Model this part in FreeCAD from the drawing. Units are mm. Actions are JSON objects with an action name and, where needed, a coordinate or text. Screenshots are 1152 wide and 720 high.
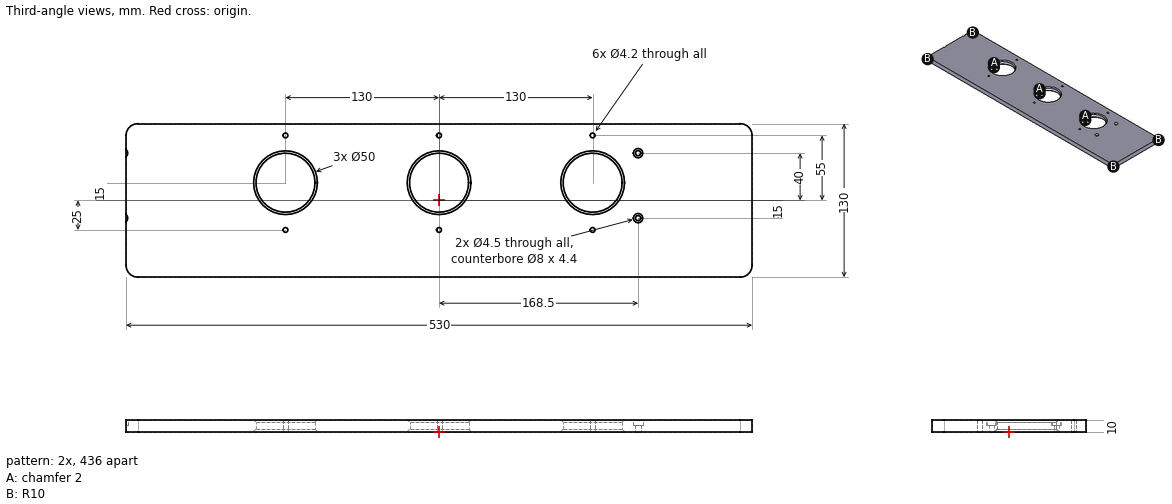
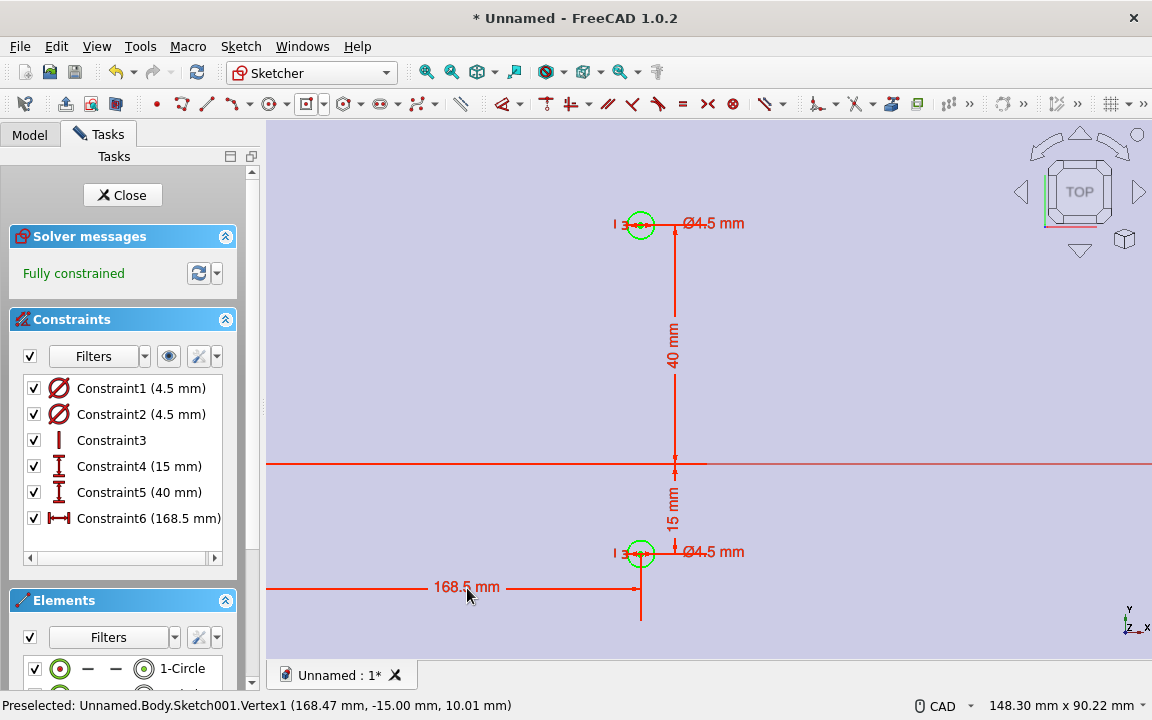
{"action": "left_click", "coordinate": [123, 195]}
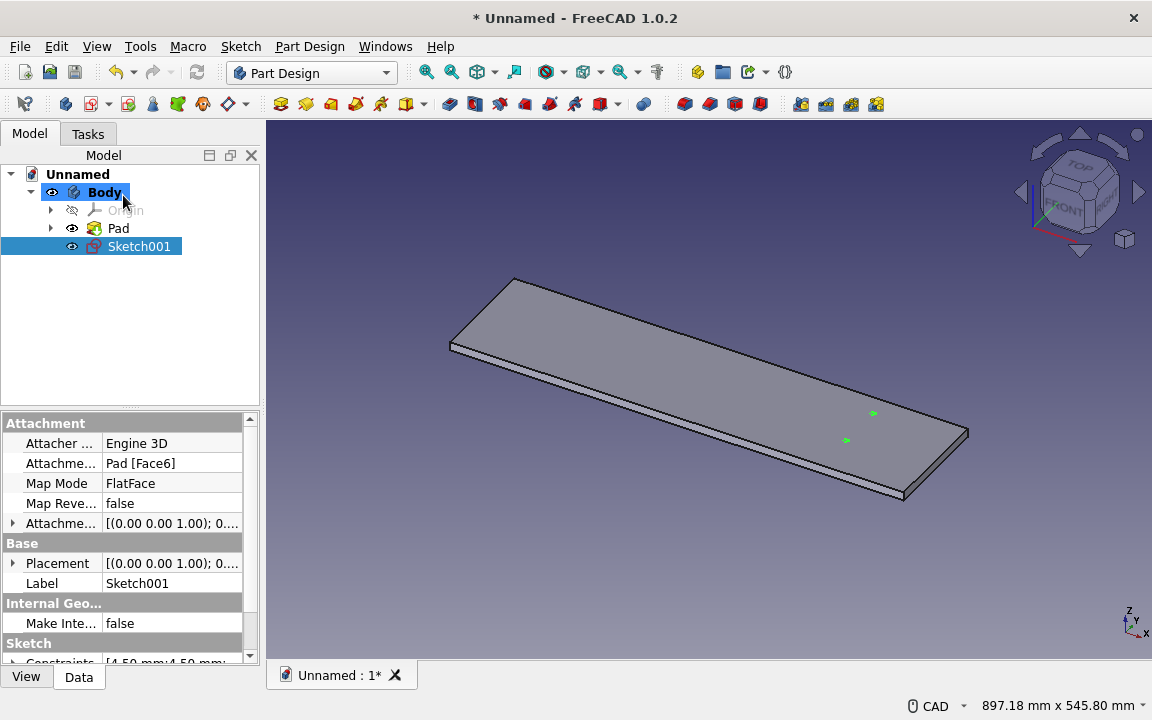
{"action": "left_click", "coordinate": [475, 104]}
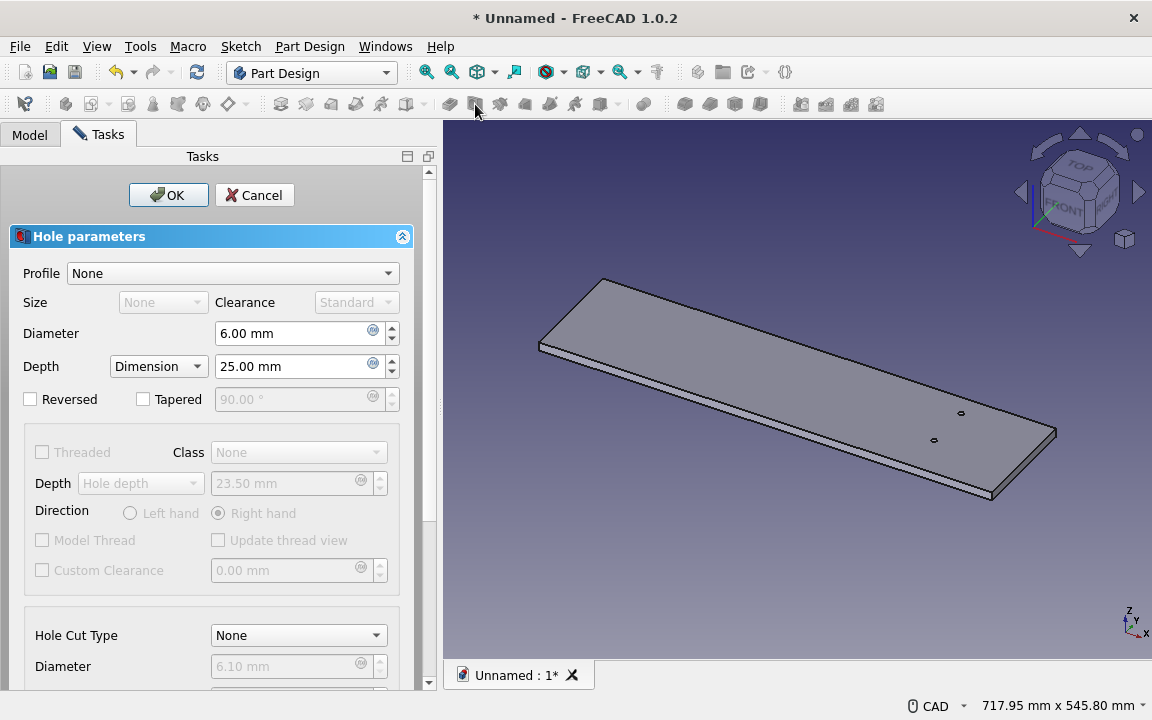
{"action": "triple_click", "coordinate": [300, 334]}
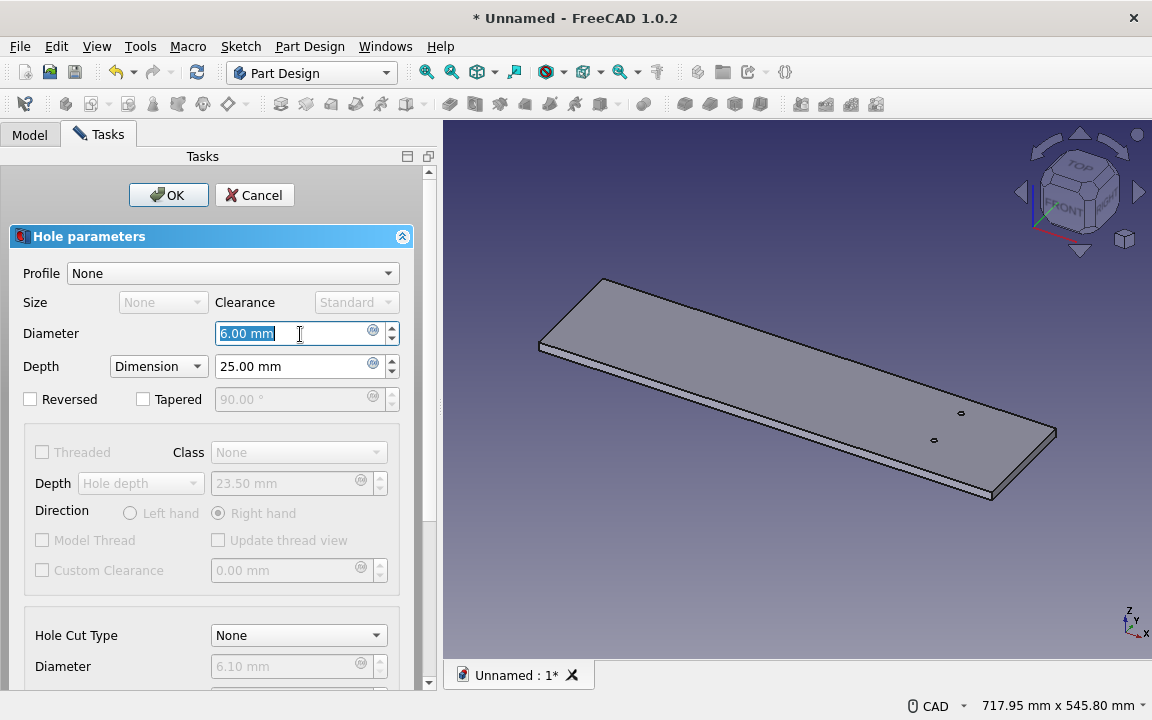
{"action": "type", "text": "4.5"}
{"action": "key", "text": "Tab"}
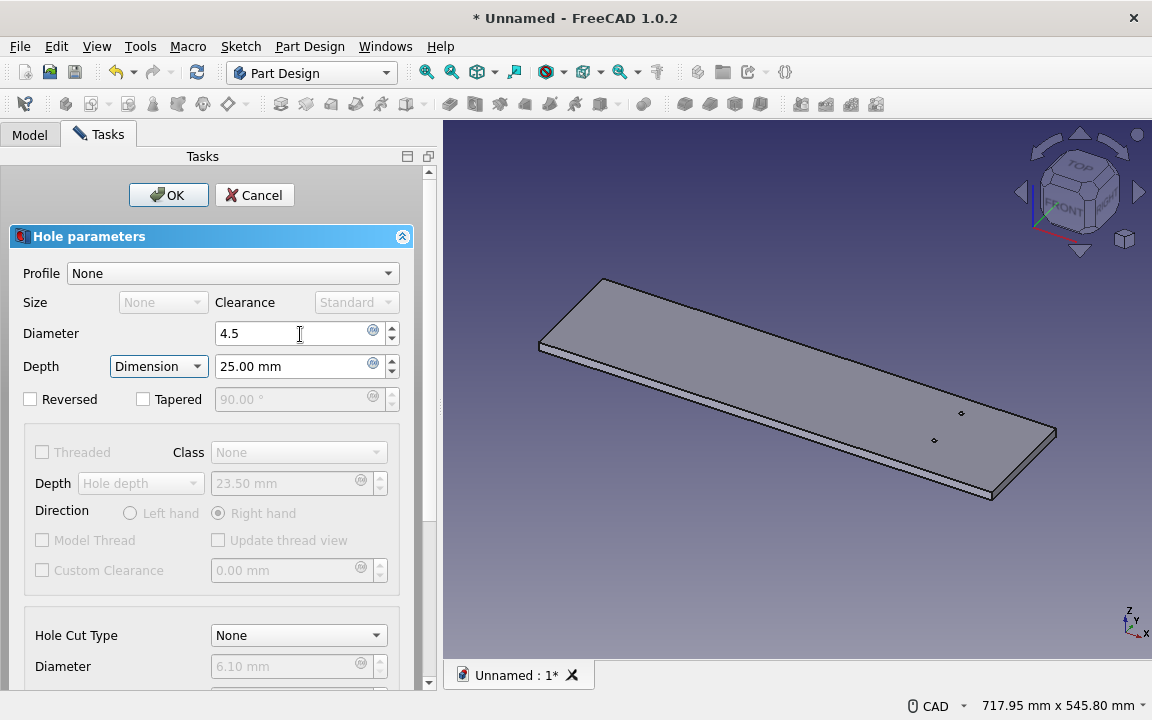
{"action": "left_click", "coordinate": [160, 366]}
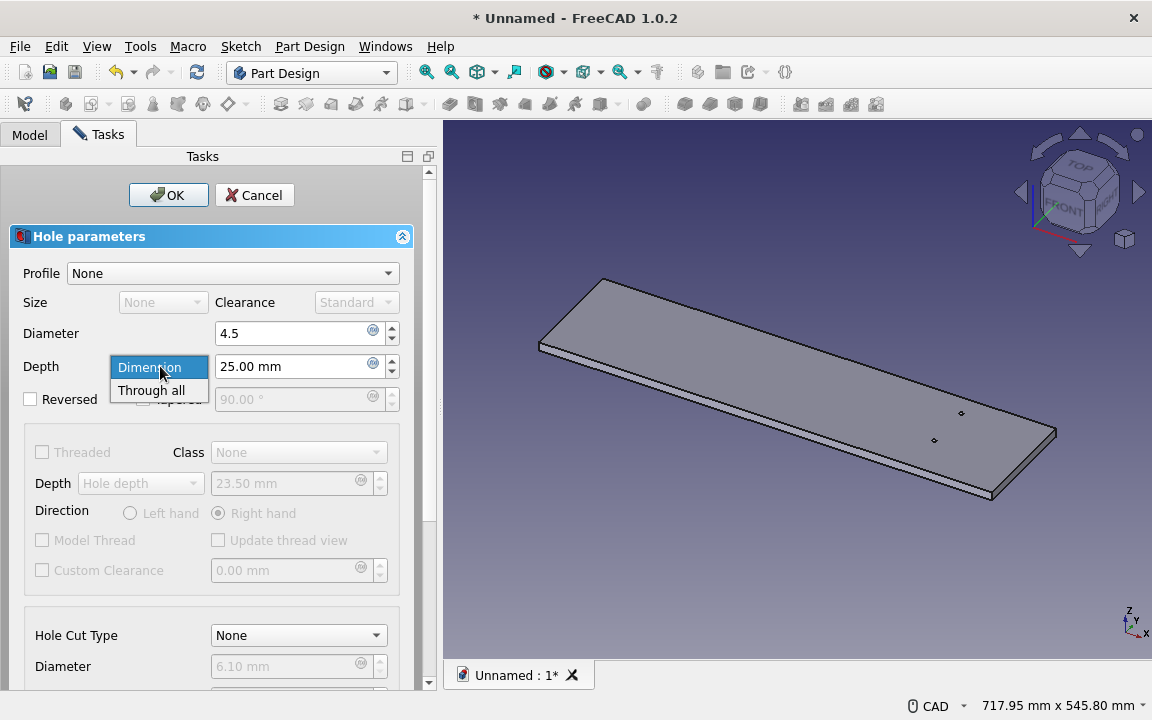
{"action": "left_click", "coordinate": [158, 390]}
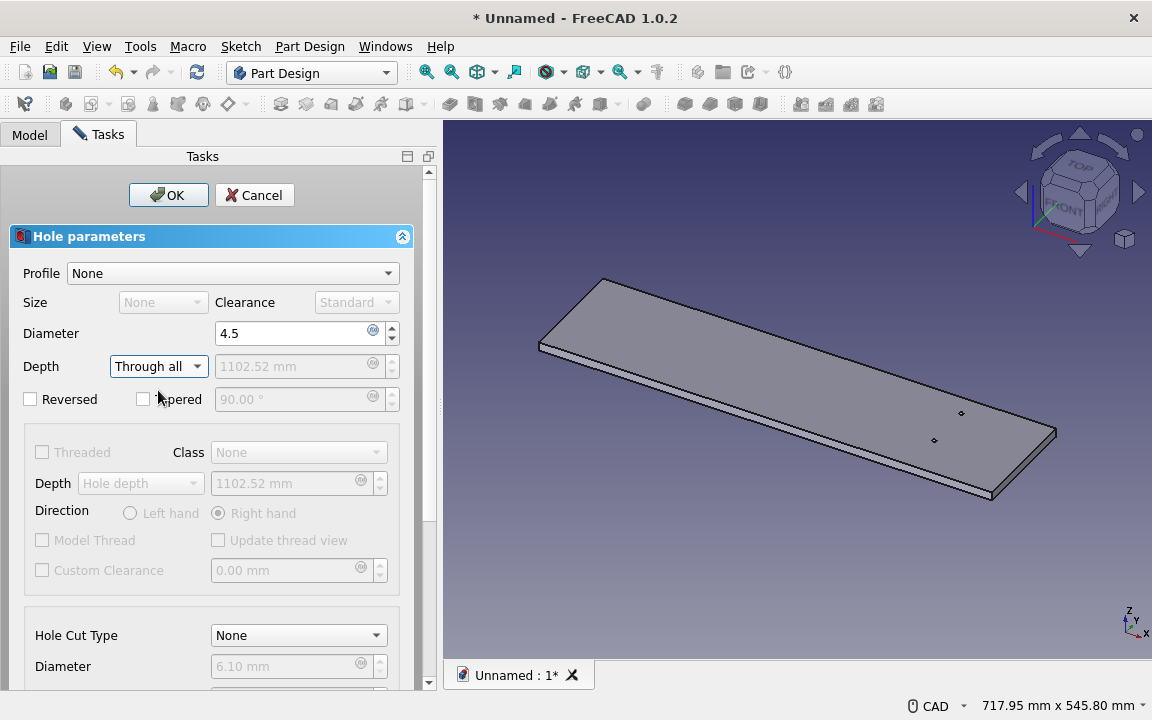
{"action": "left_click", "coordinate": [300, 636]}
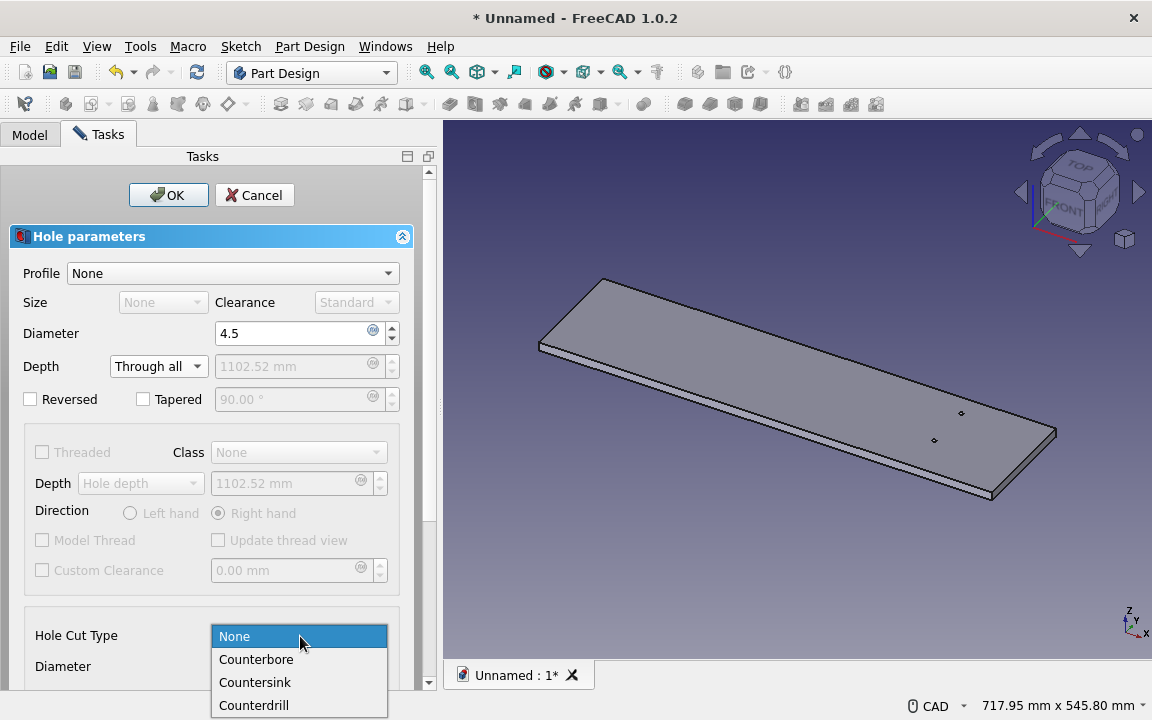
{"action": "left_click", "coordinate": [298, 660]}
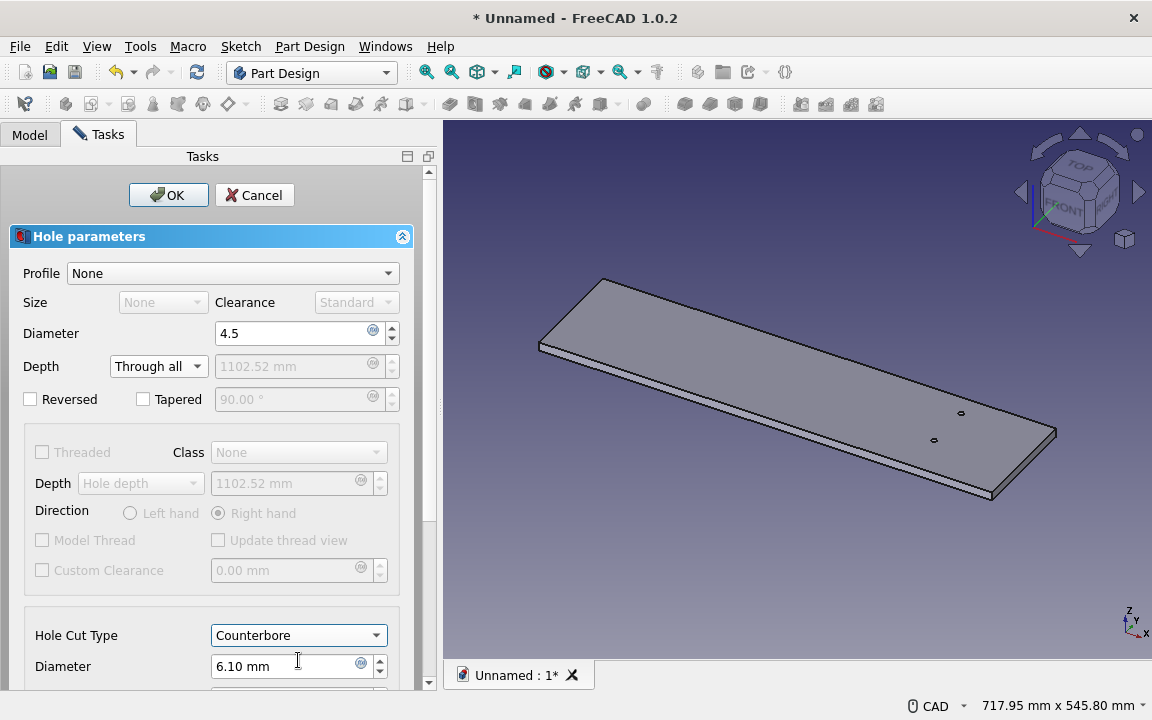
{"action": "triple_click", "coordinate": [292, 666]}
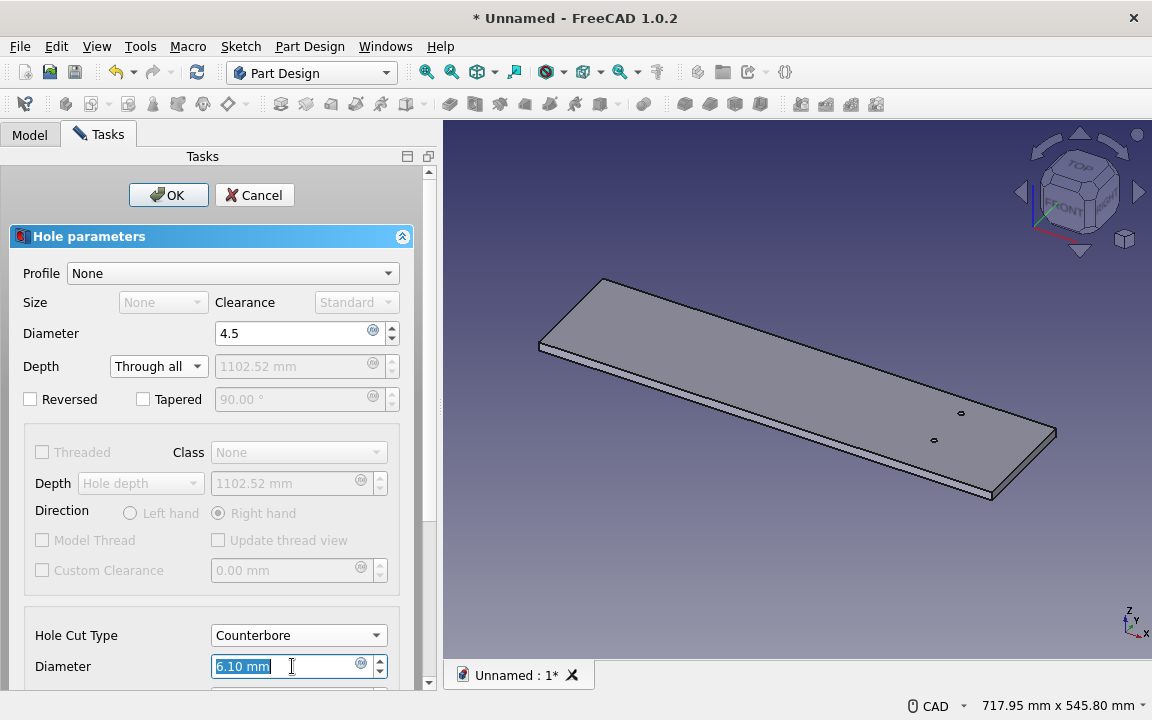
{"action": "type", "text": "8"}
{"action": "key", "text": "Tab"}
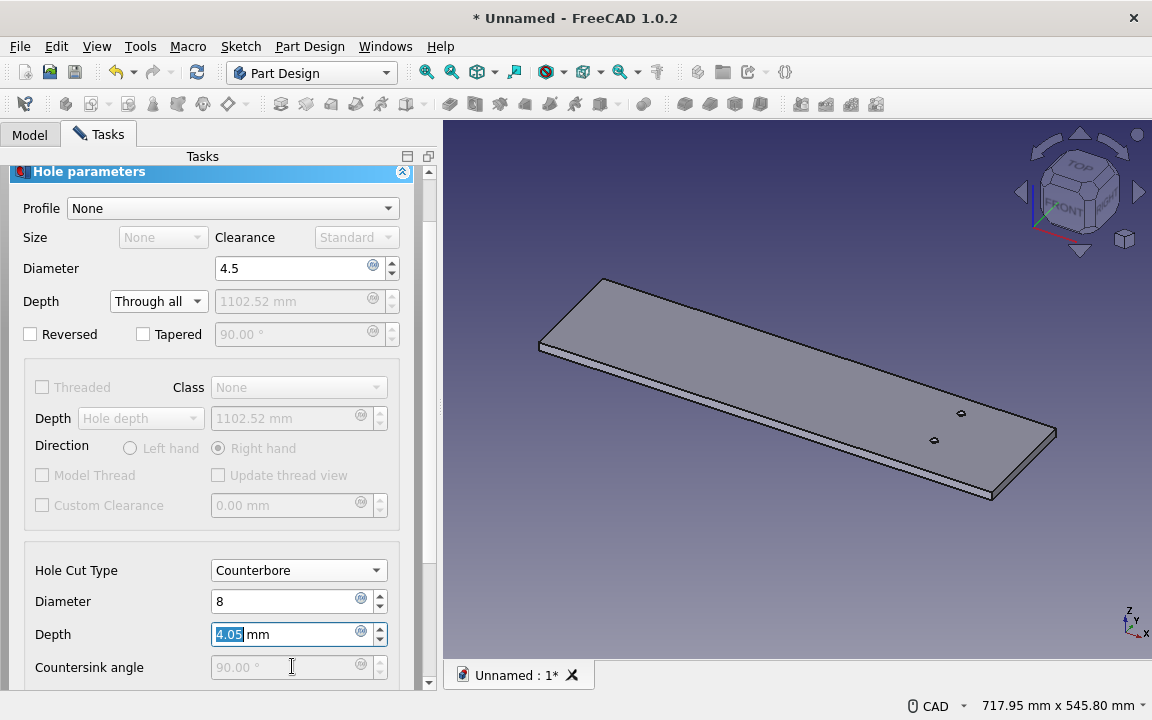
{"action": "type", "text": "4.4"}
{"action": "key", "text": "Tab"}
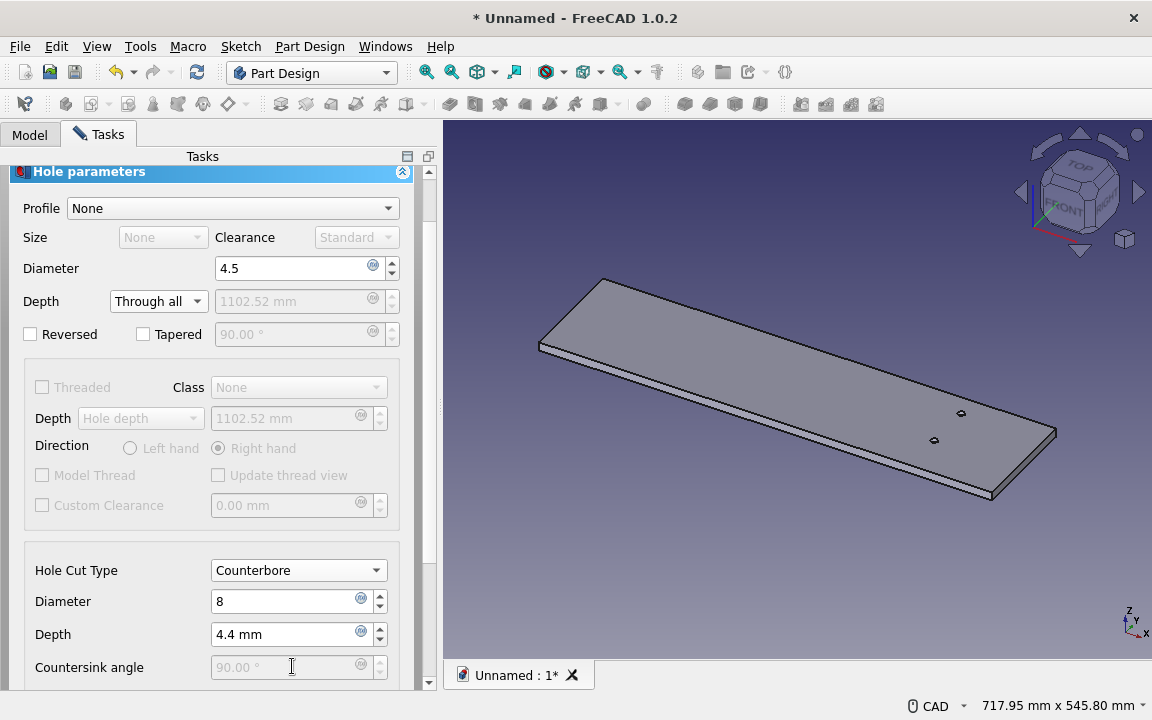
{"action": "scroll", "coordinate": [429, 428], "scroll_direction": "up", "scroll_amount": 2}